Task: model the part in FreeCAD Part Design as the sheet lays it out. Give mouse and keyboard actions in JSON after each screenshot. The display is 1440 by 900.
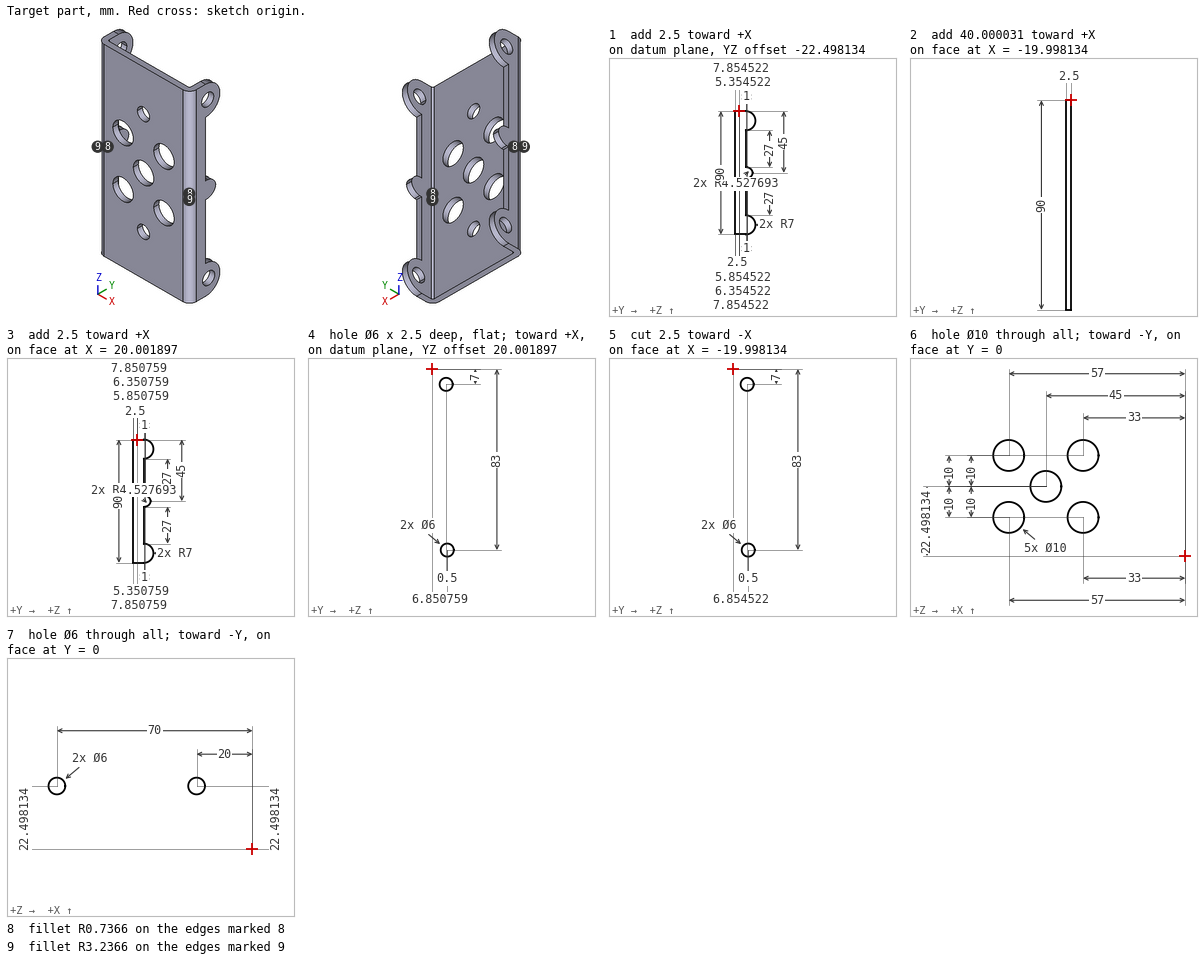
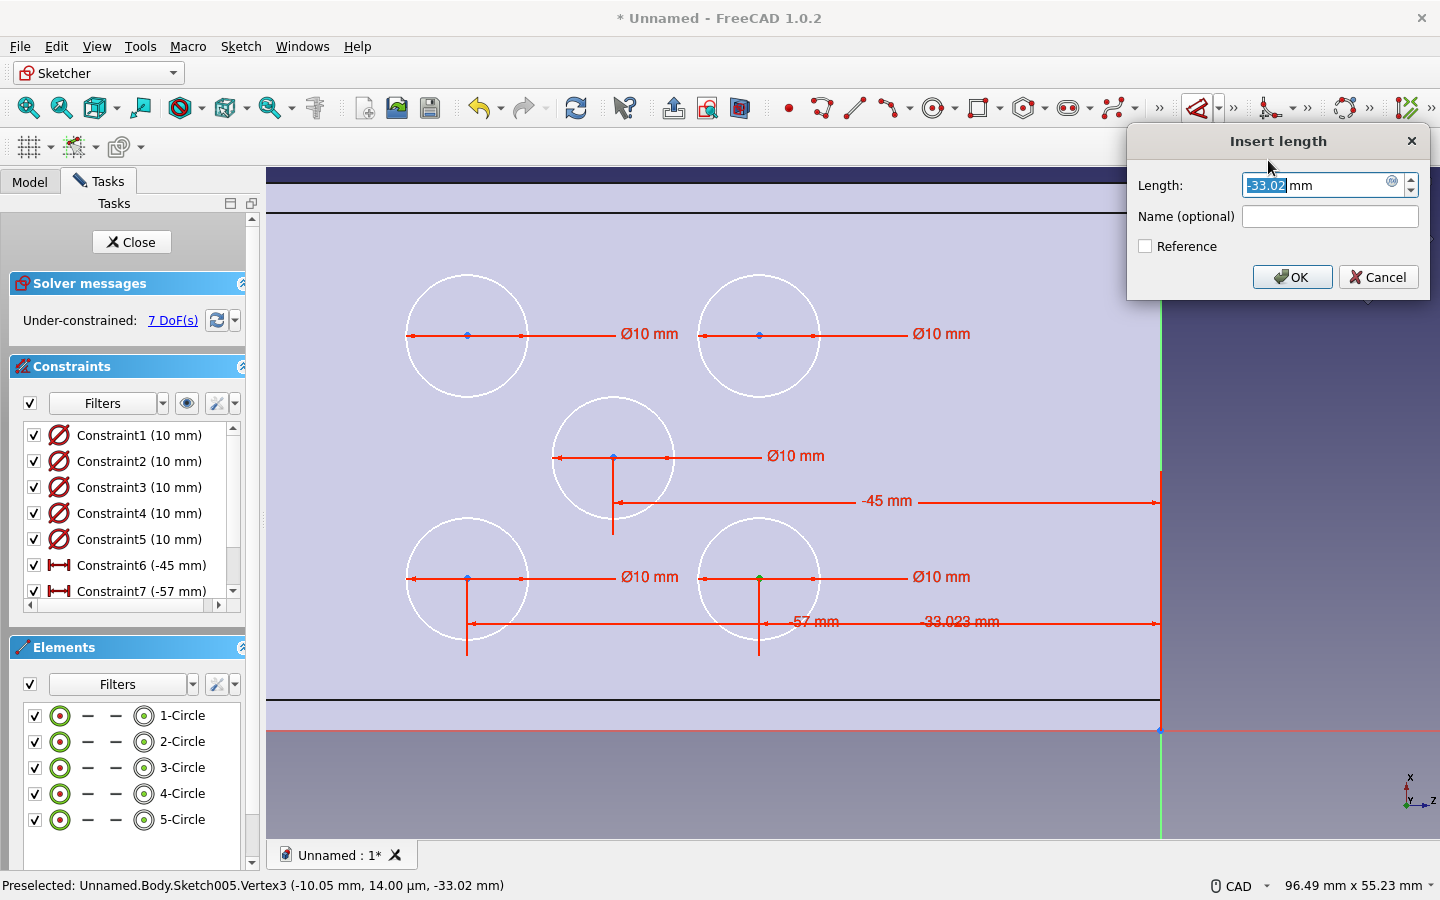
{"action": "type", "text": "-33"}
{"action": "key", "text": "Return"}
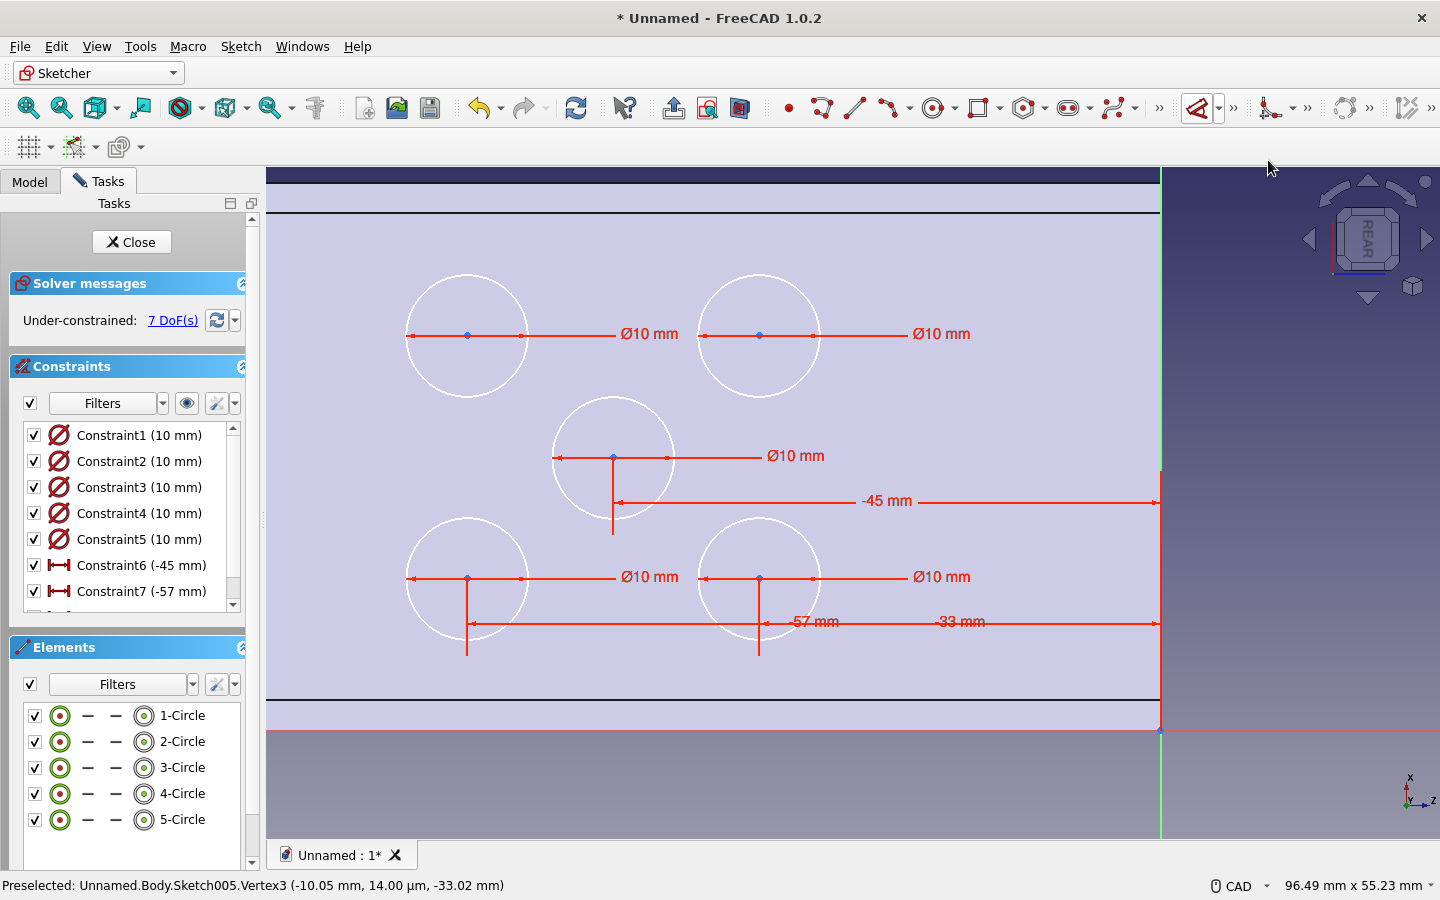
{"action": "left_click", "coordinate": [759, 336]}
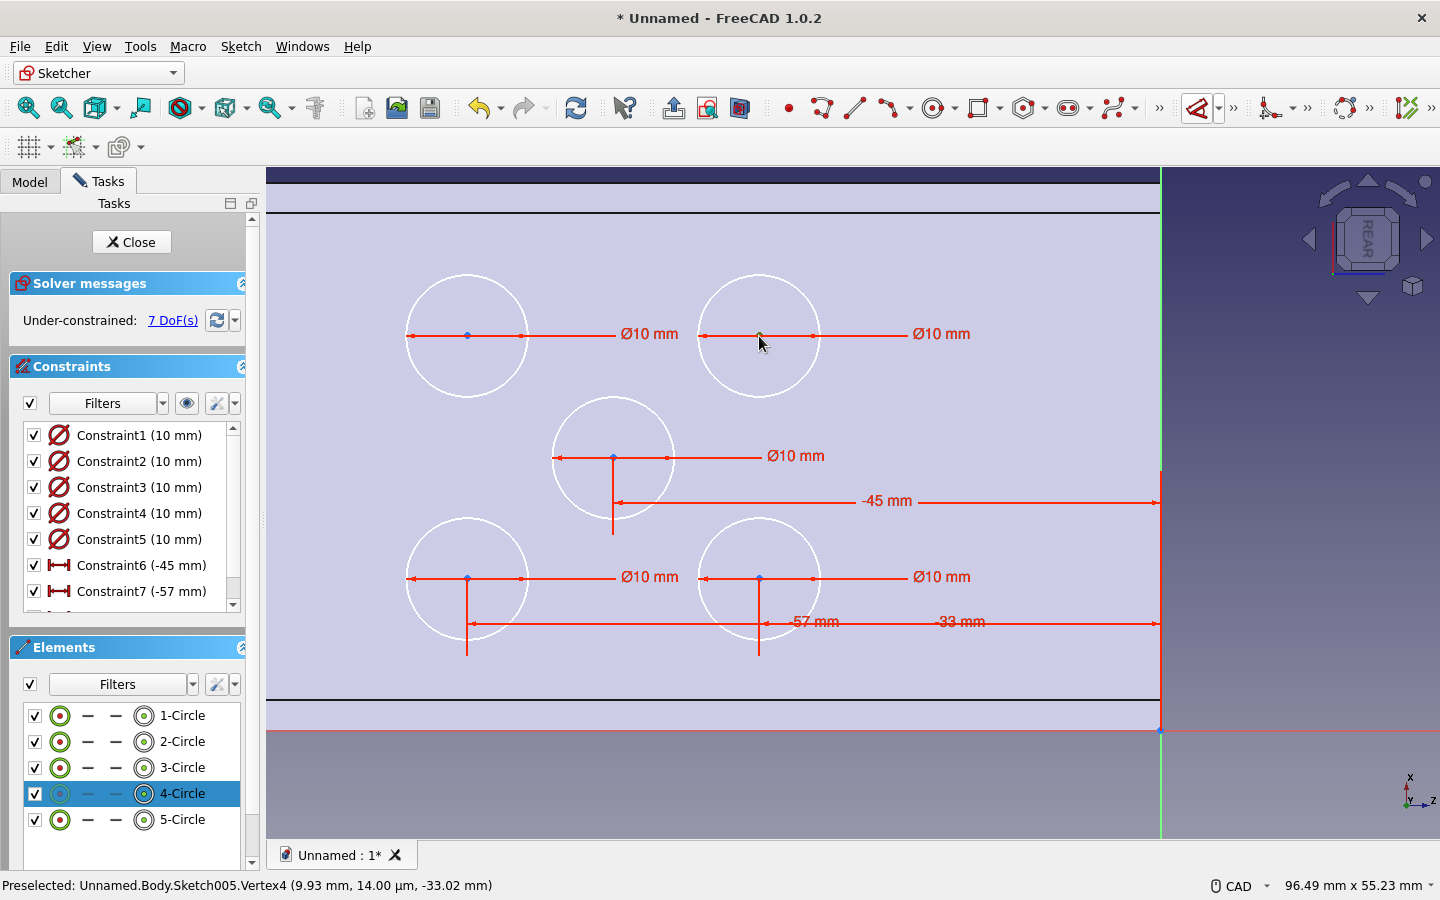
{"action": "key", "text": "l"}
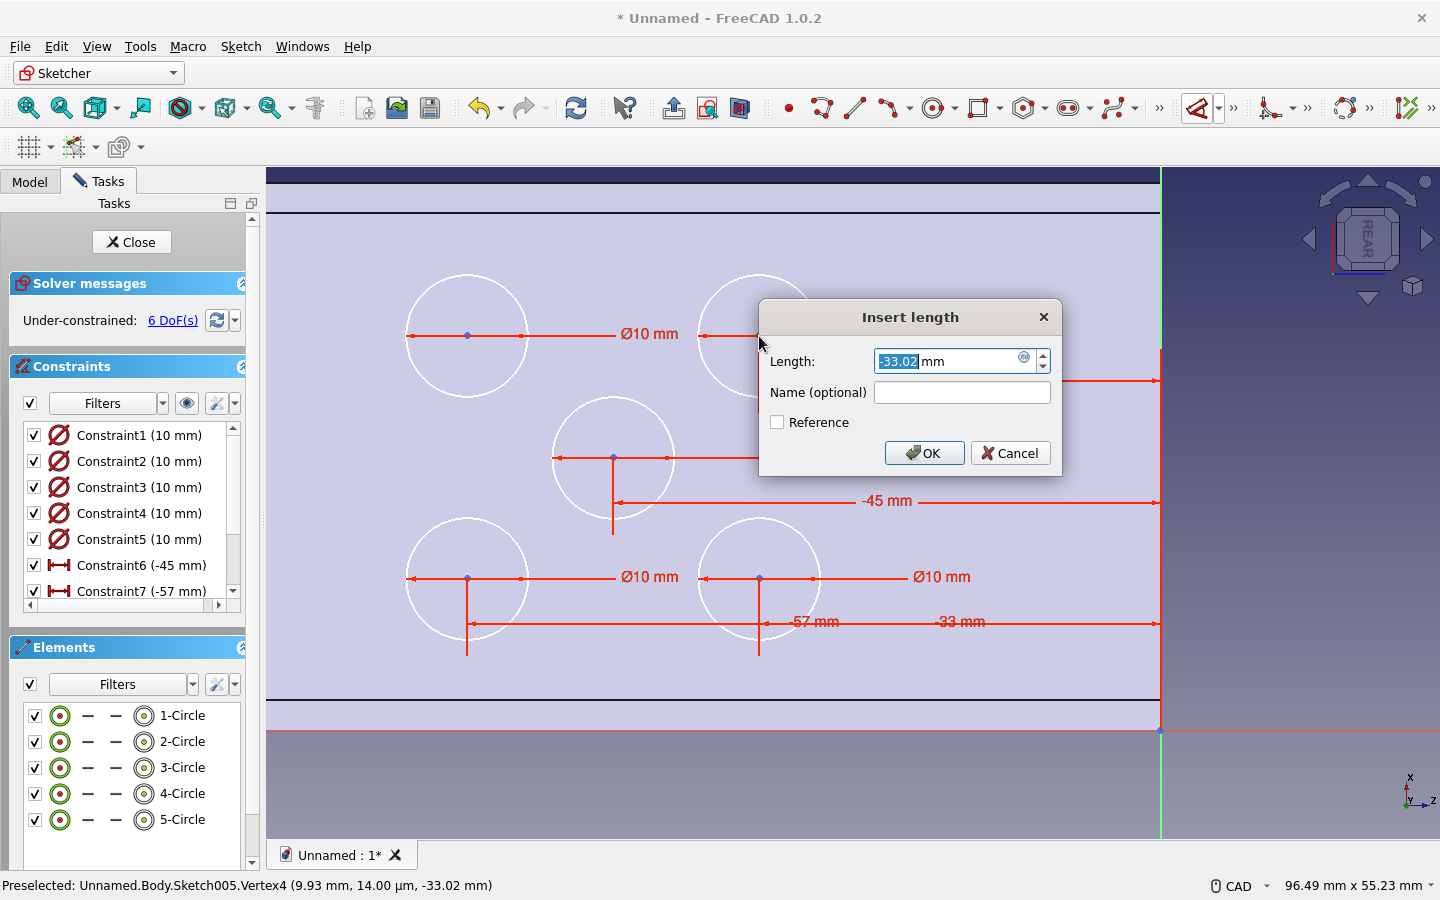
{"action": "type", "text": "-33"}
{"action": "key", "text": "Return"}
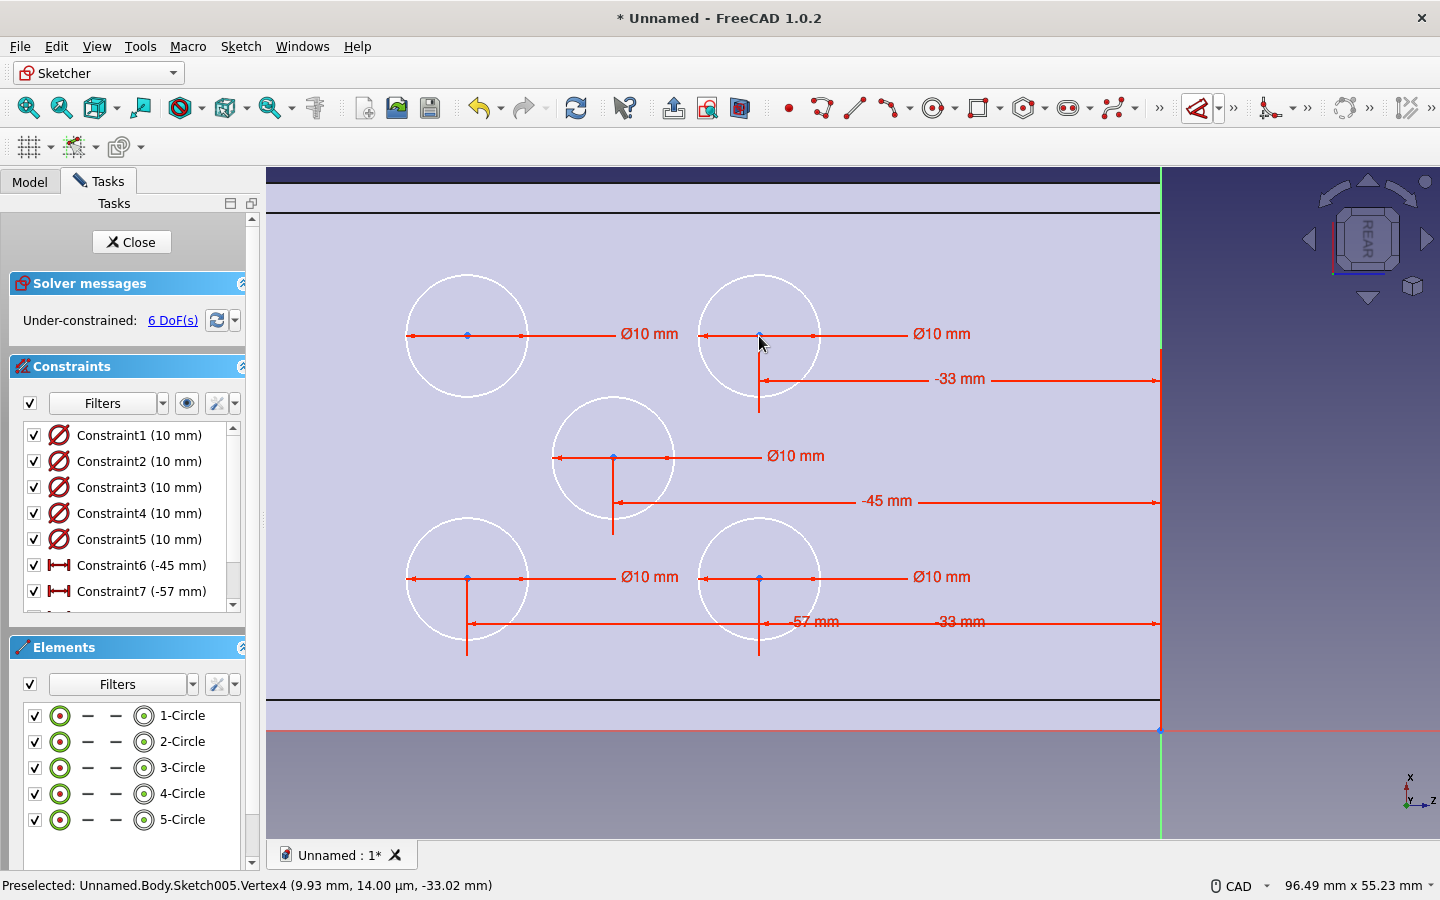
{"action": "left_click", "coordinate": [467, 336]}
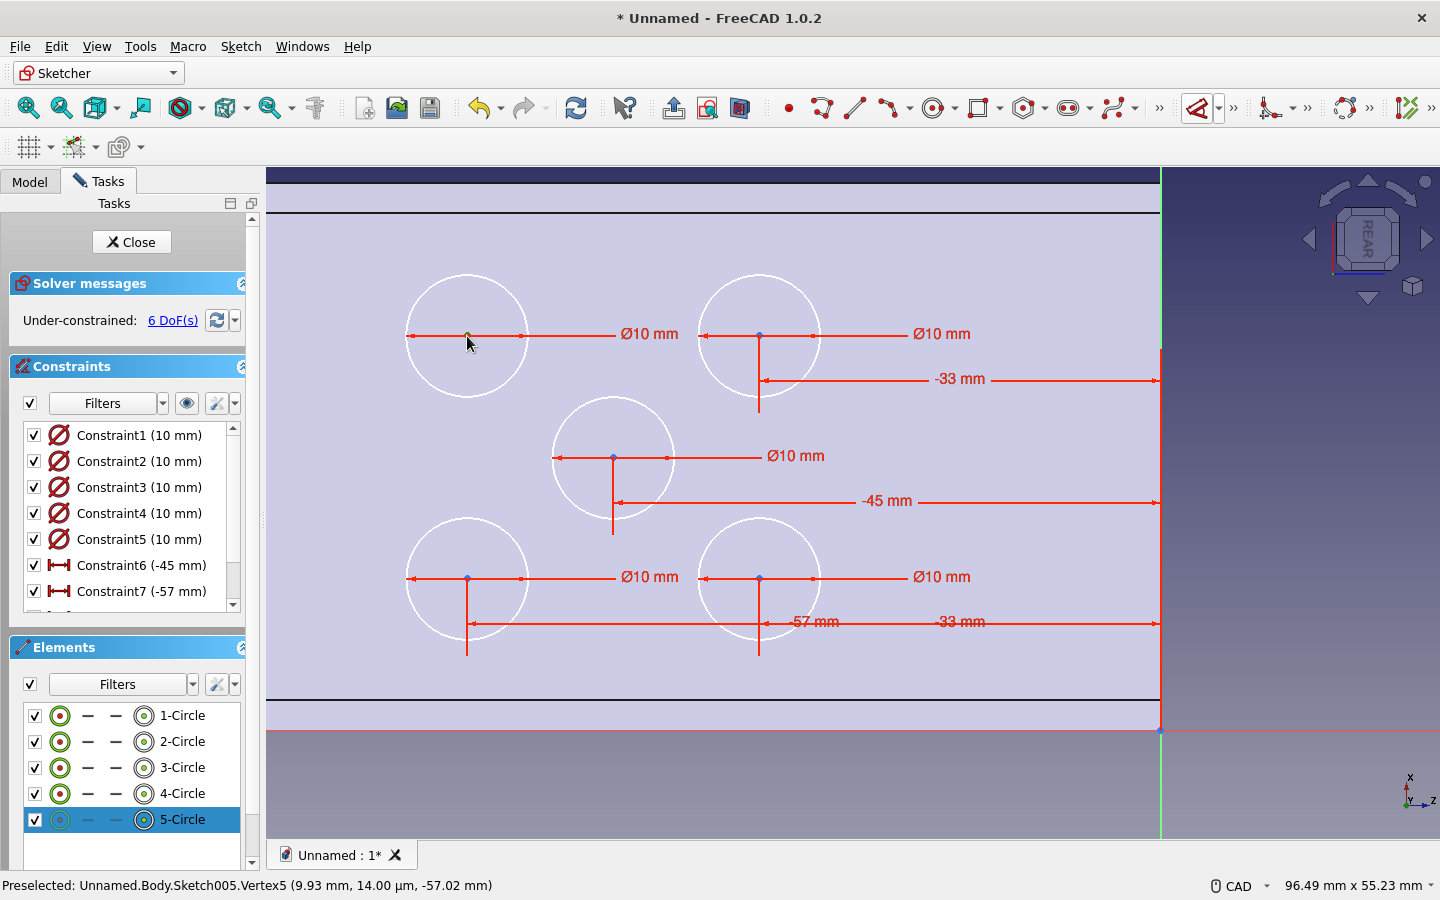
{"action": "key", "text": "l"}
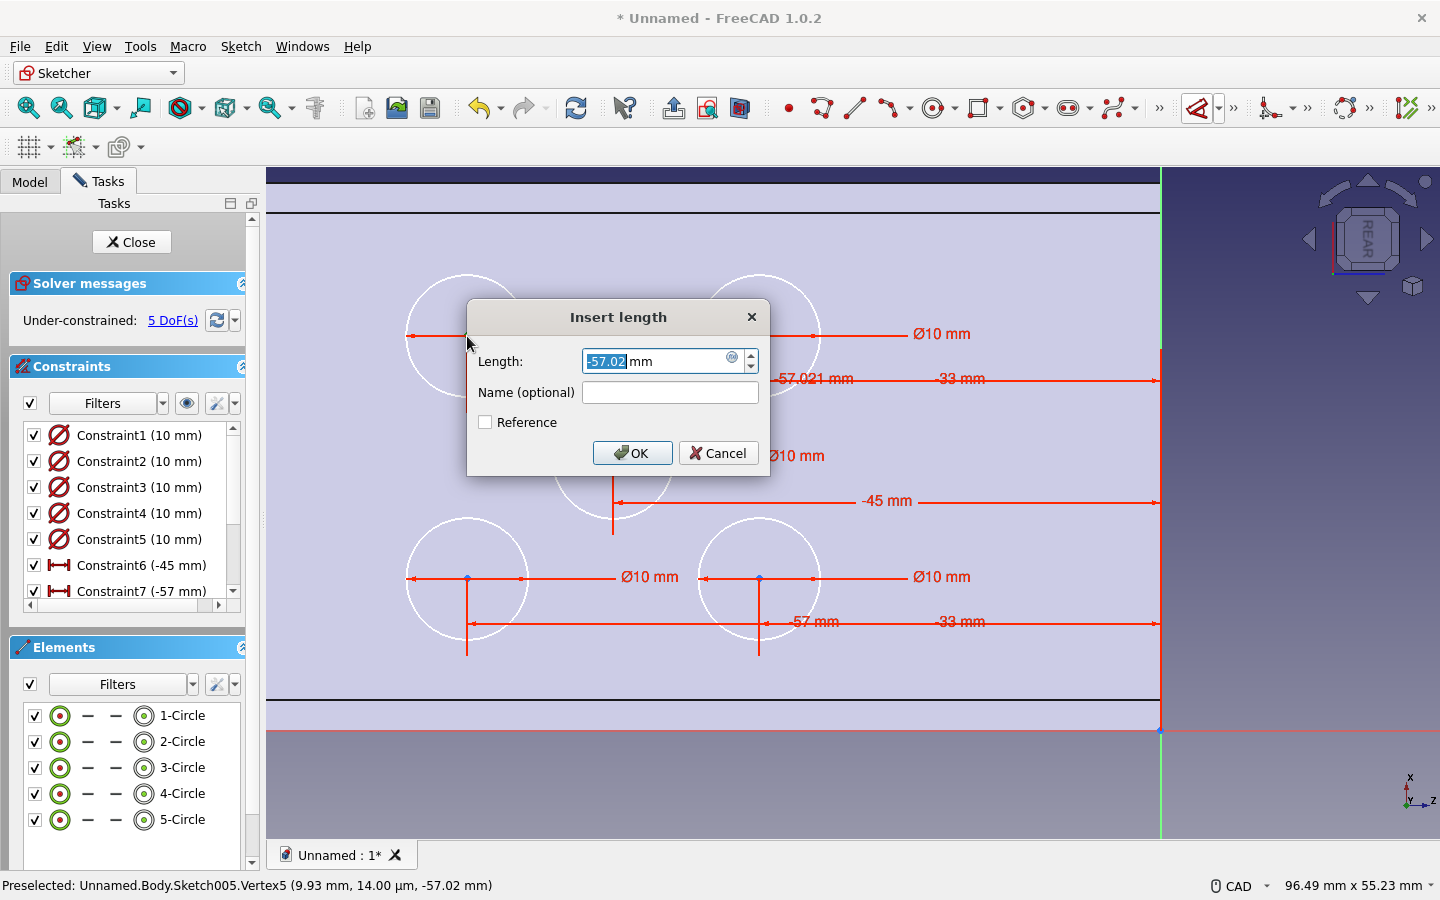
{"action": "type", "text": "-57"}
{"action": "key", "text": "Return"}